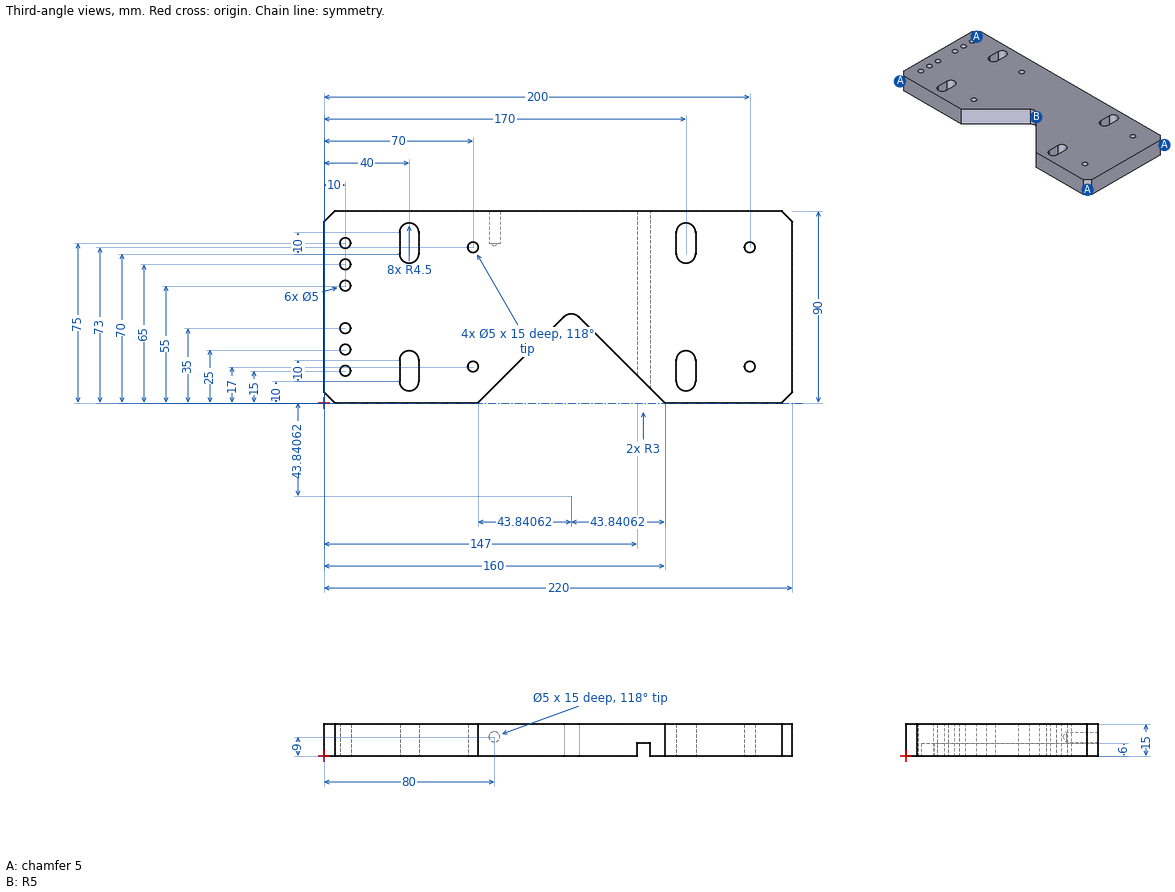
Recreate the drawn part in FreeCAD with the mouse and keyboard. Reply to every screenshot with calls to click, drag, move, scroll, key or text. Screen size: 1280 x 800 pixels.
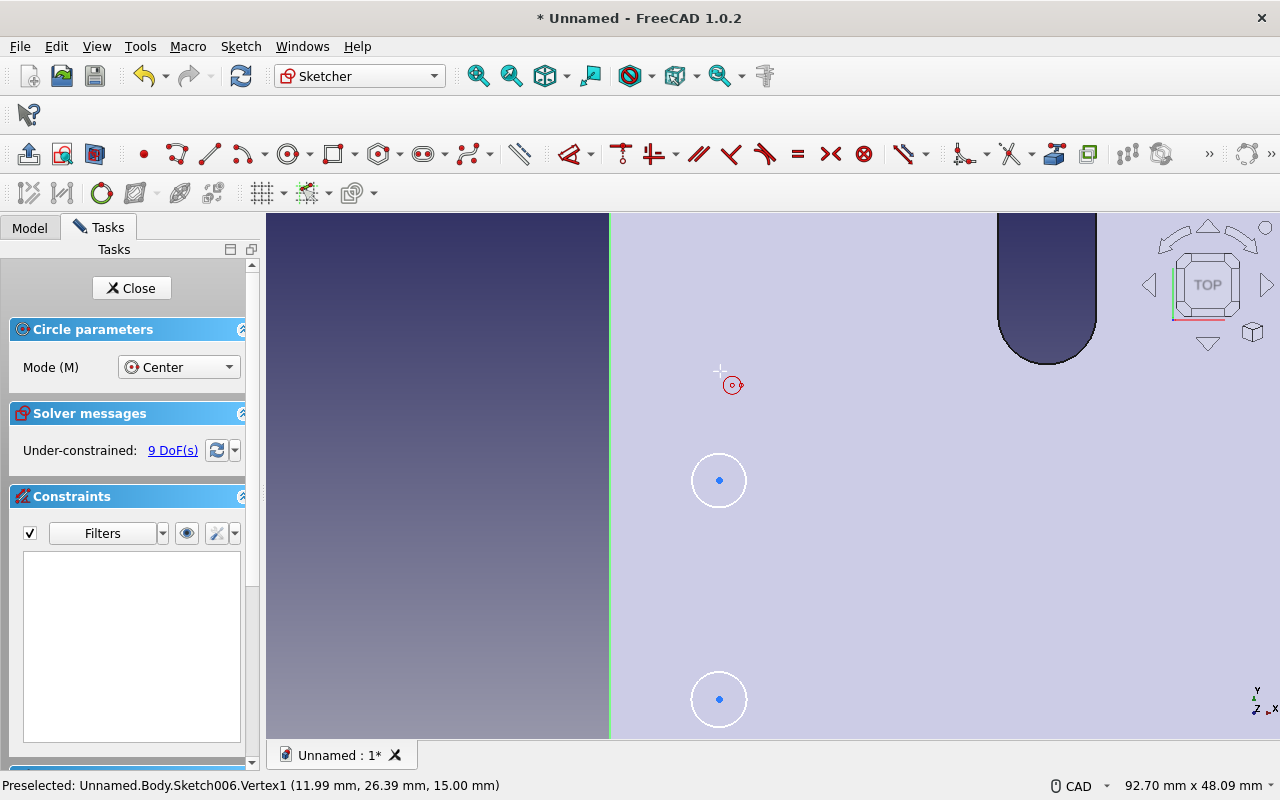
click(719, 370)
click(738, 351)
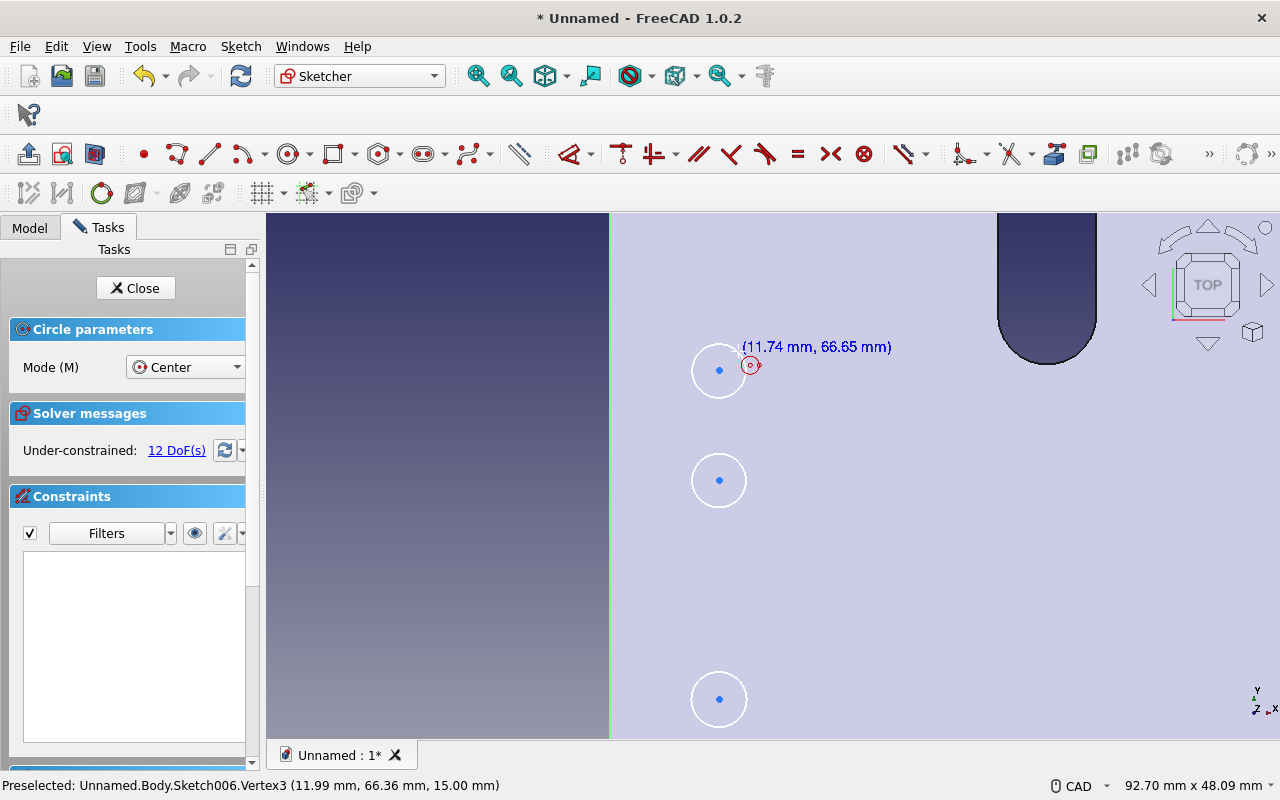
click(719, 261)
click(738, 241)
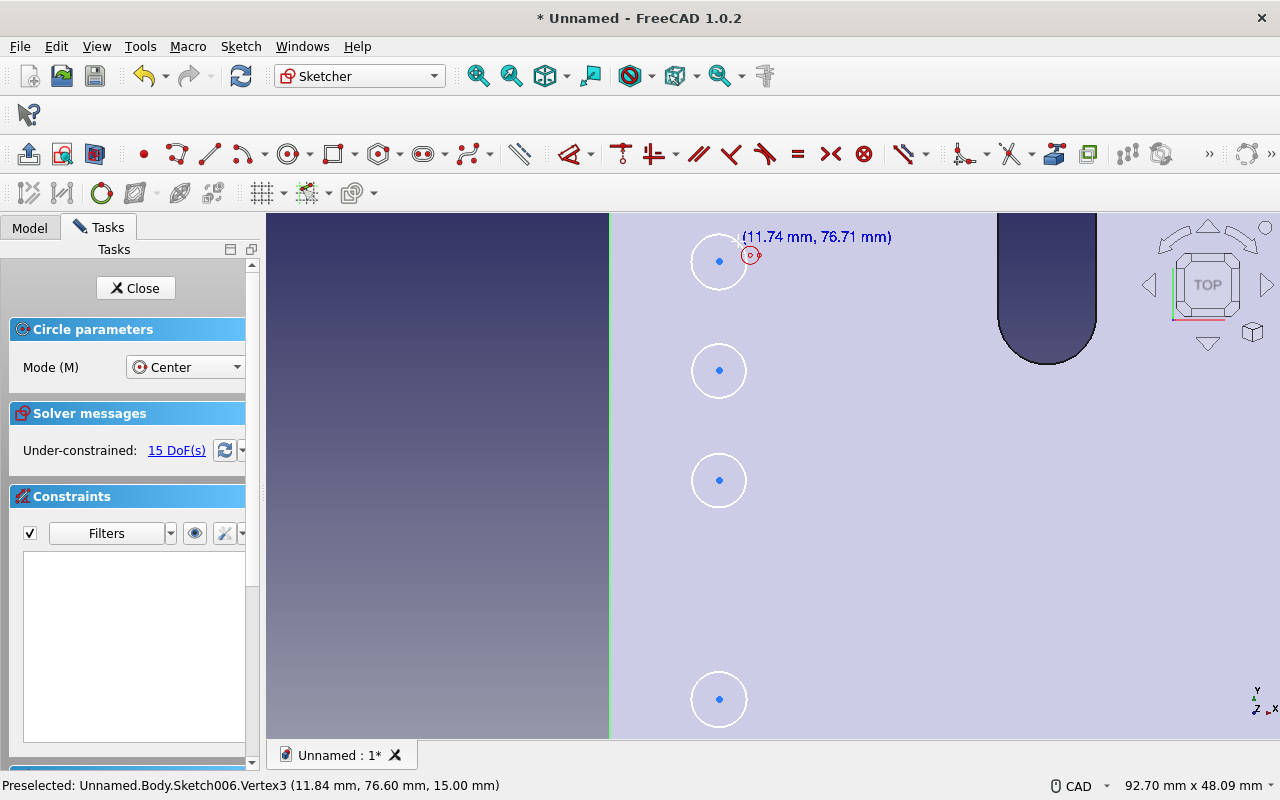
scroll(720, 371, down, 5)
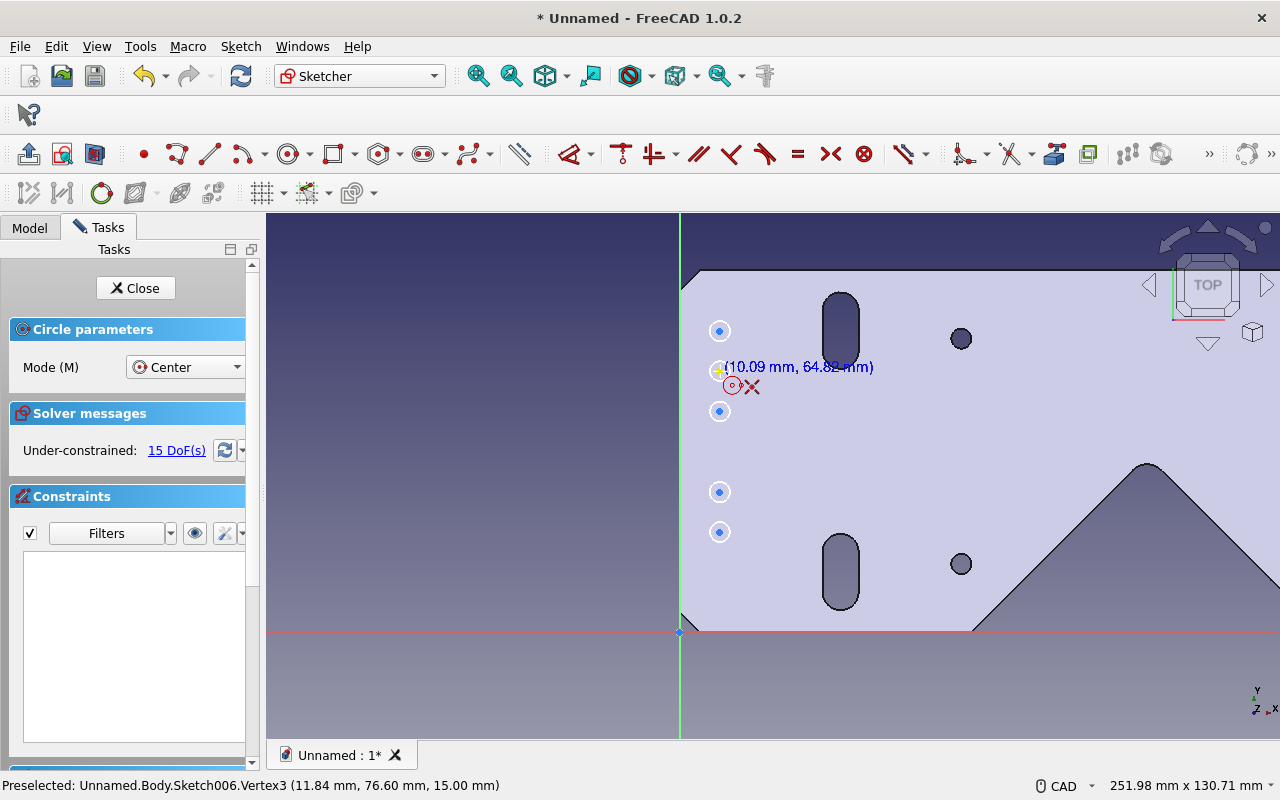
scroll(720, 572, up, 5)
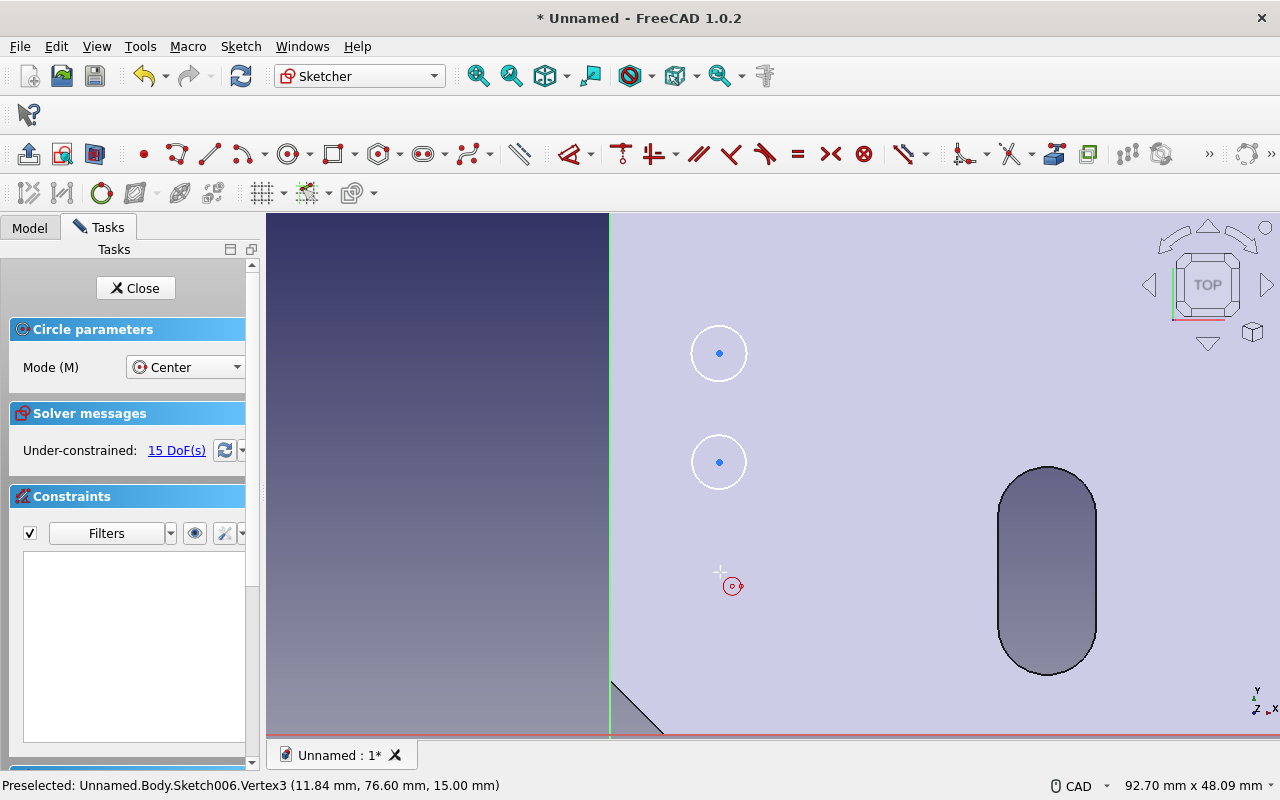
click(719, 571)
click(738, 552)
key(Escape)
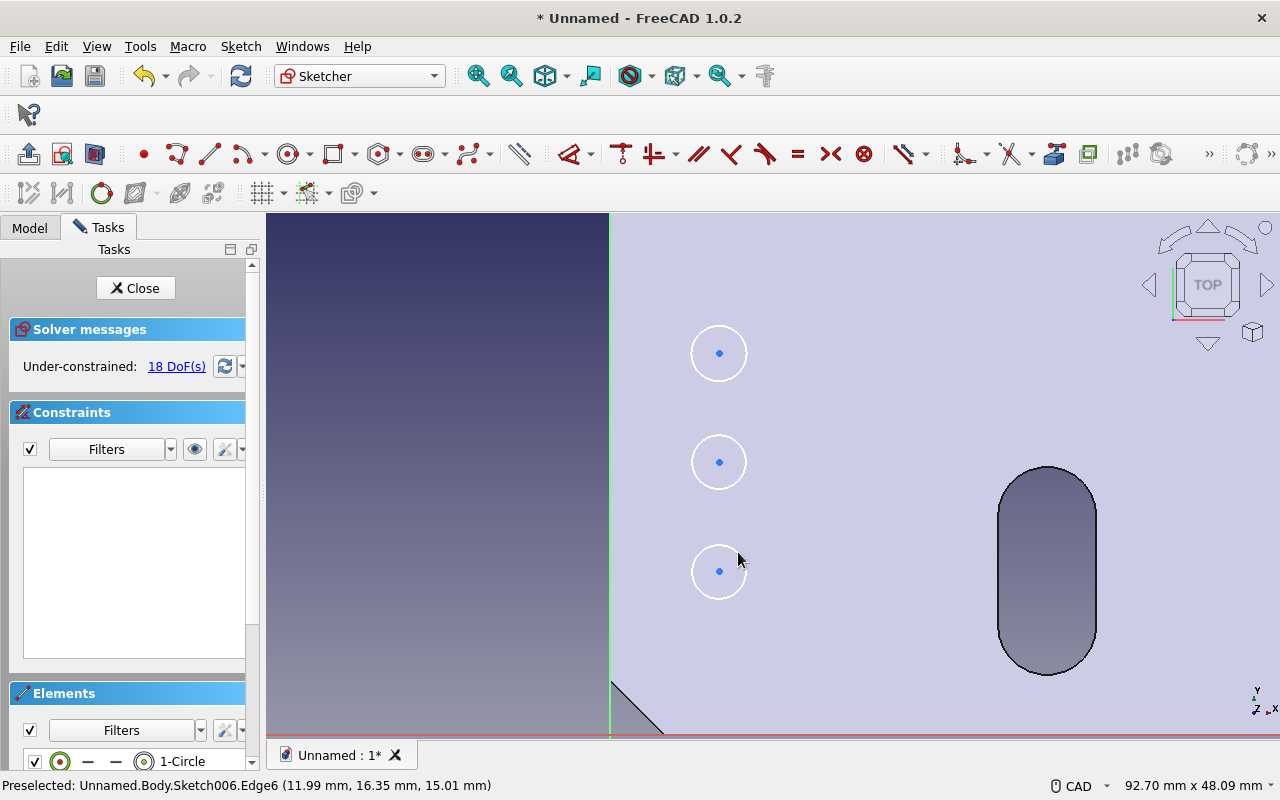
scroll(720, 572, down, 5)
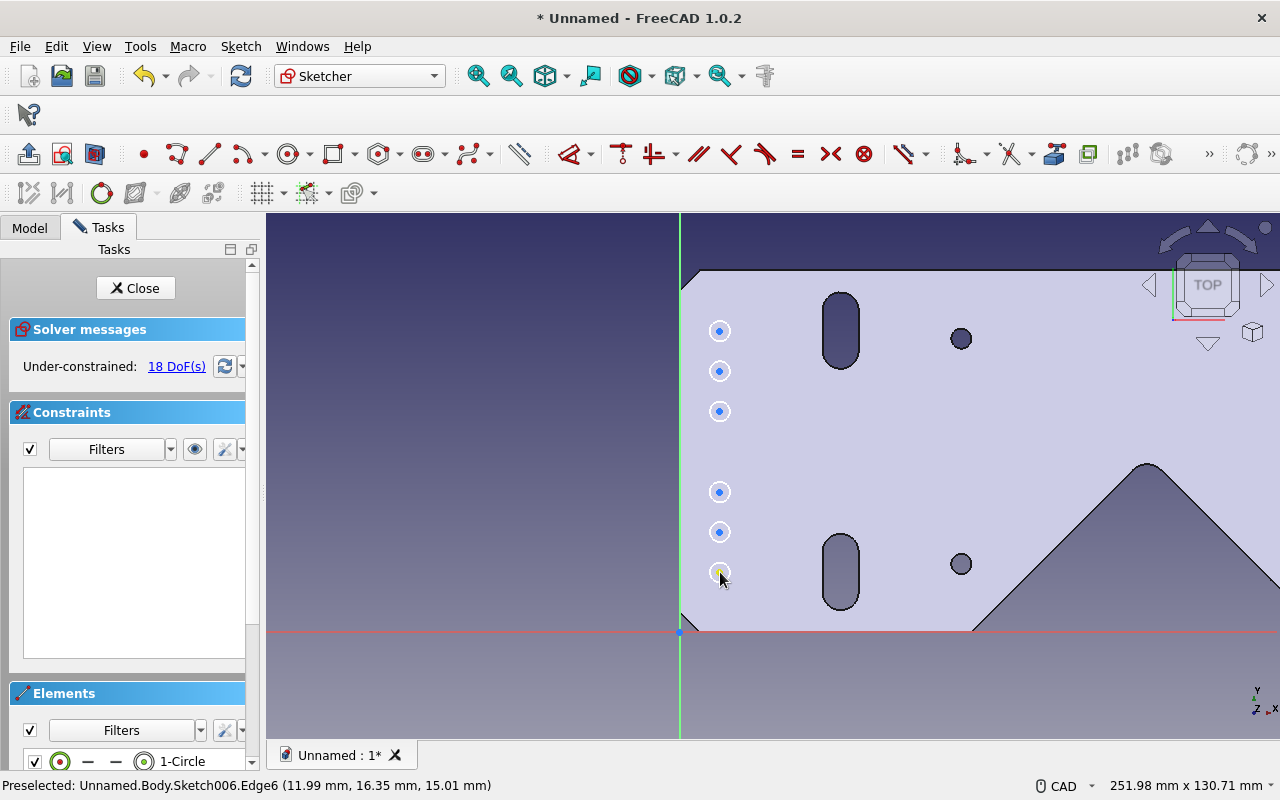
scroll(727, 404, up, 2)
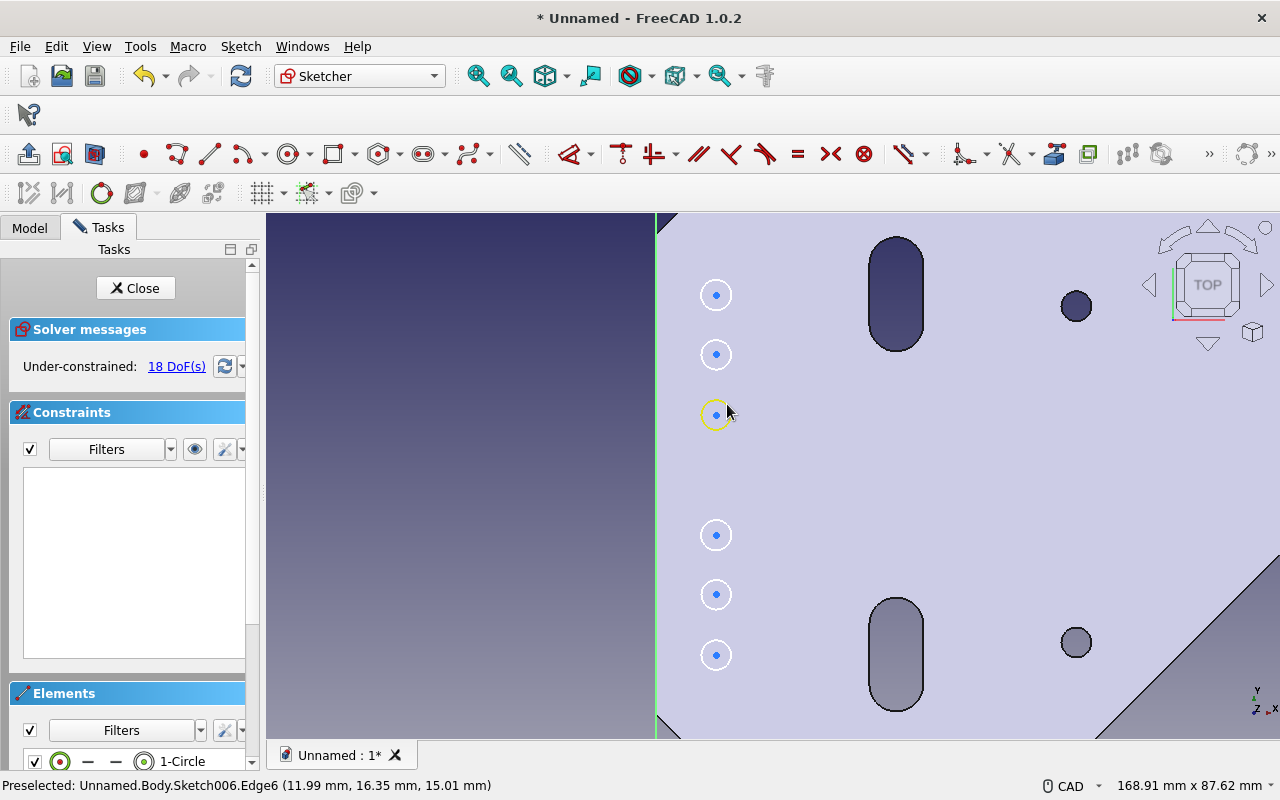
click(727, 405)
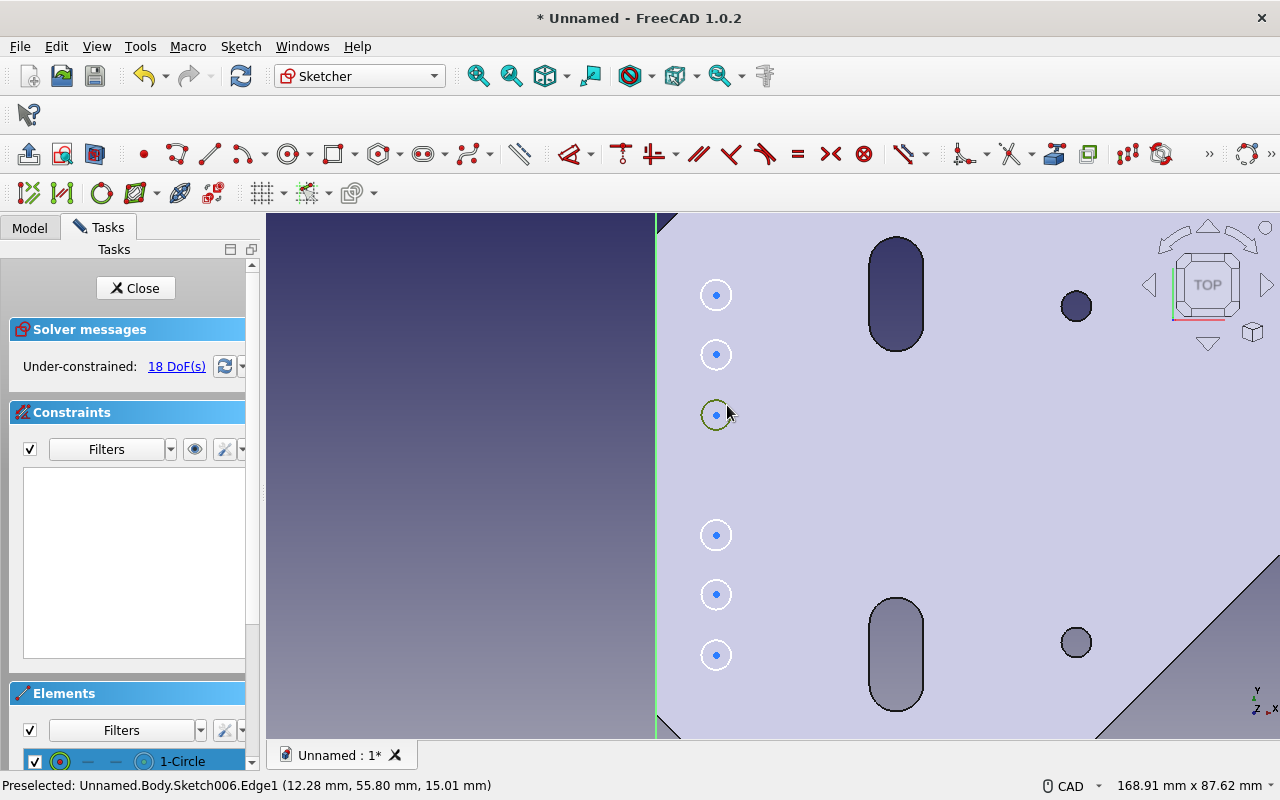
click(727, 524)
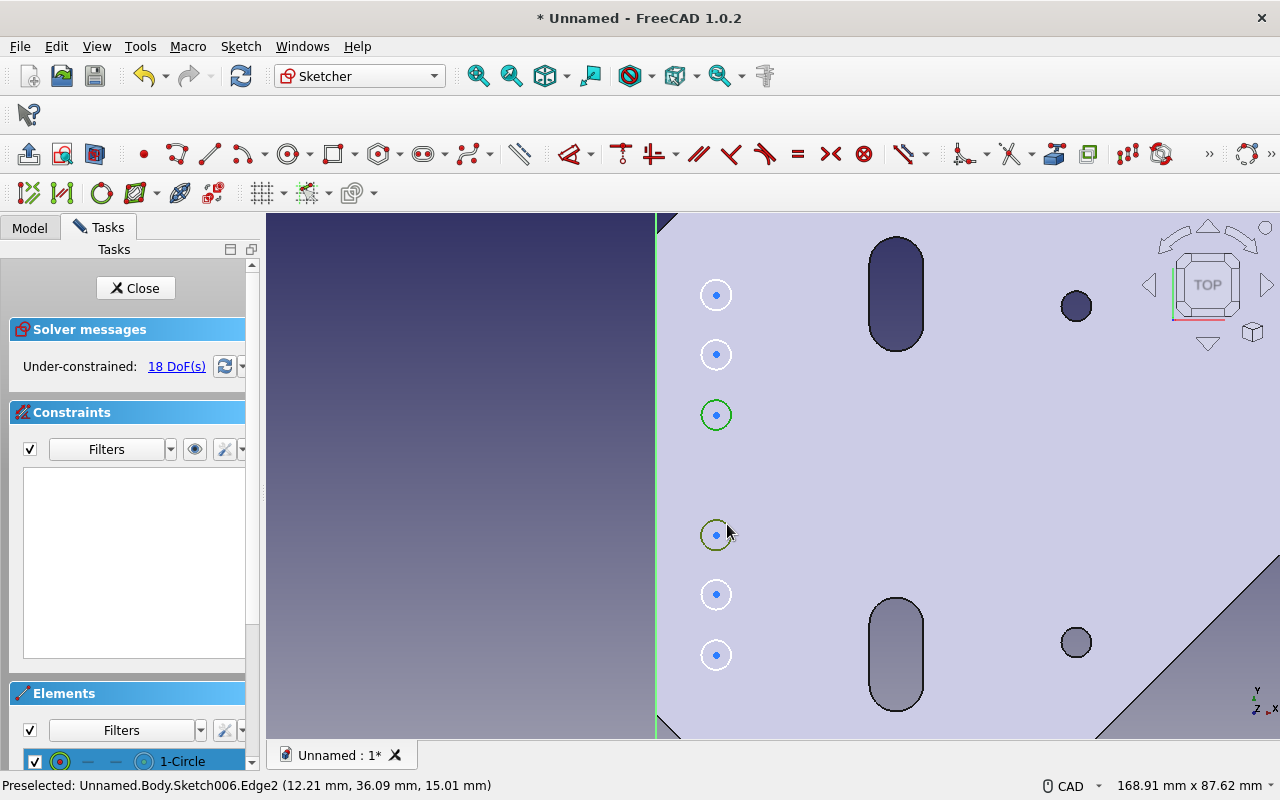
click(727, 584)